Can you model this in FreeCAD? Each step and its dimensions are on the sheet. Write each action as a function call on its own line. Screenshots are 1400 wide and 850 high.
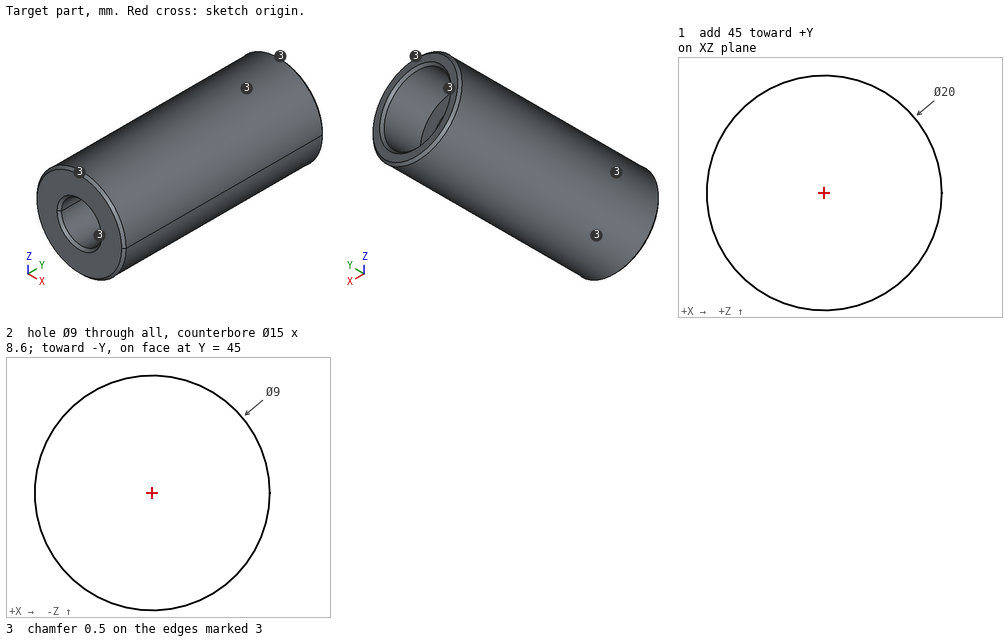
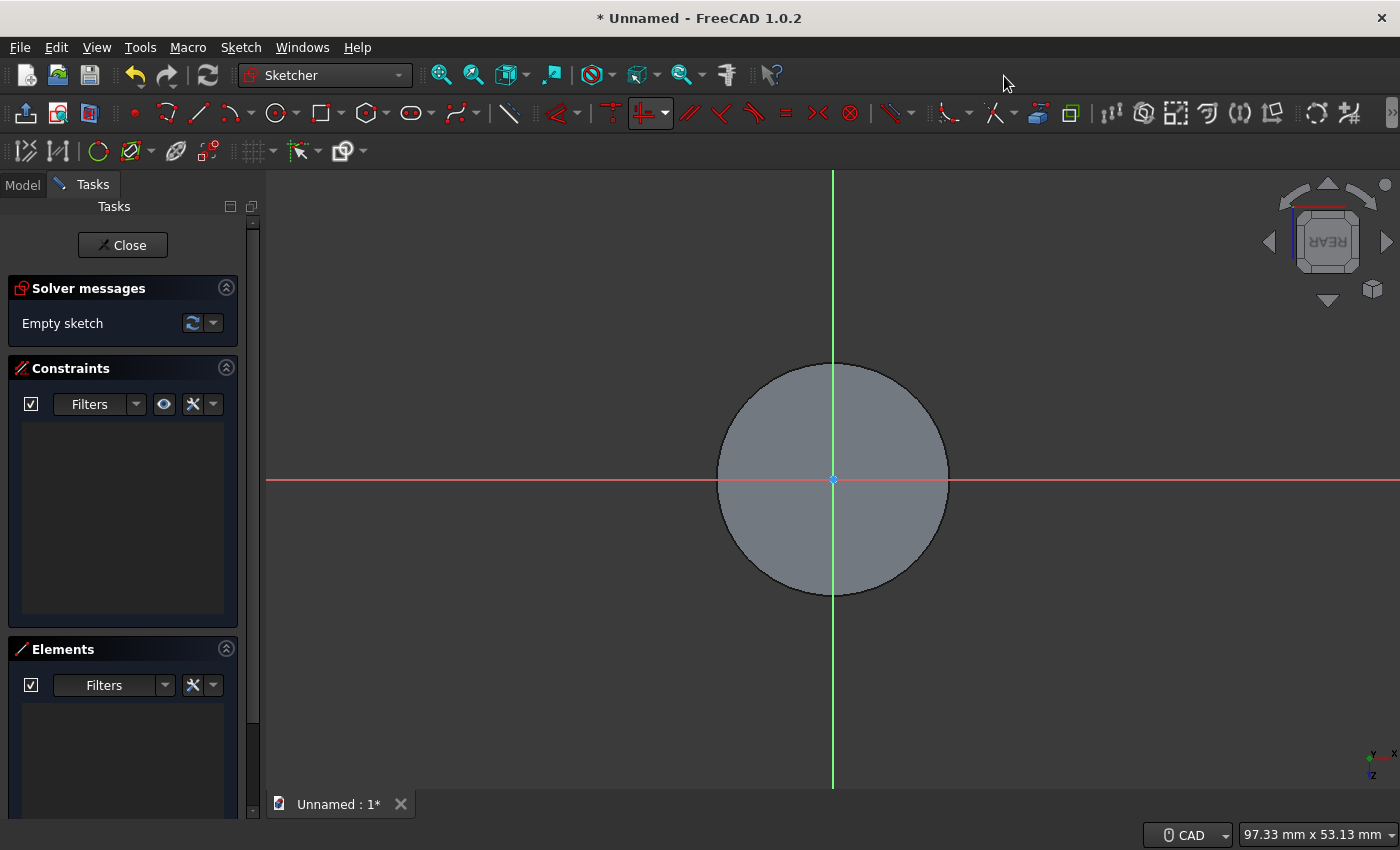
scroll(855, 479, up, 7)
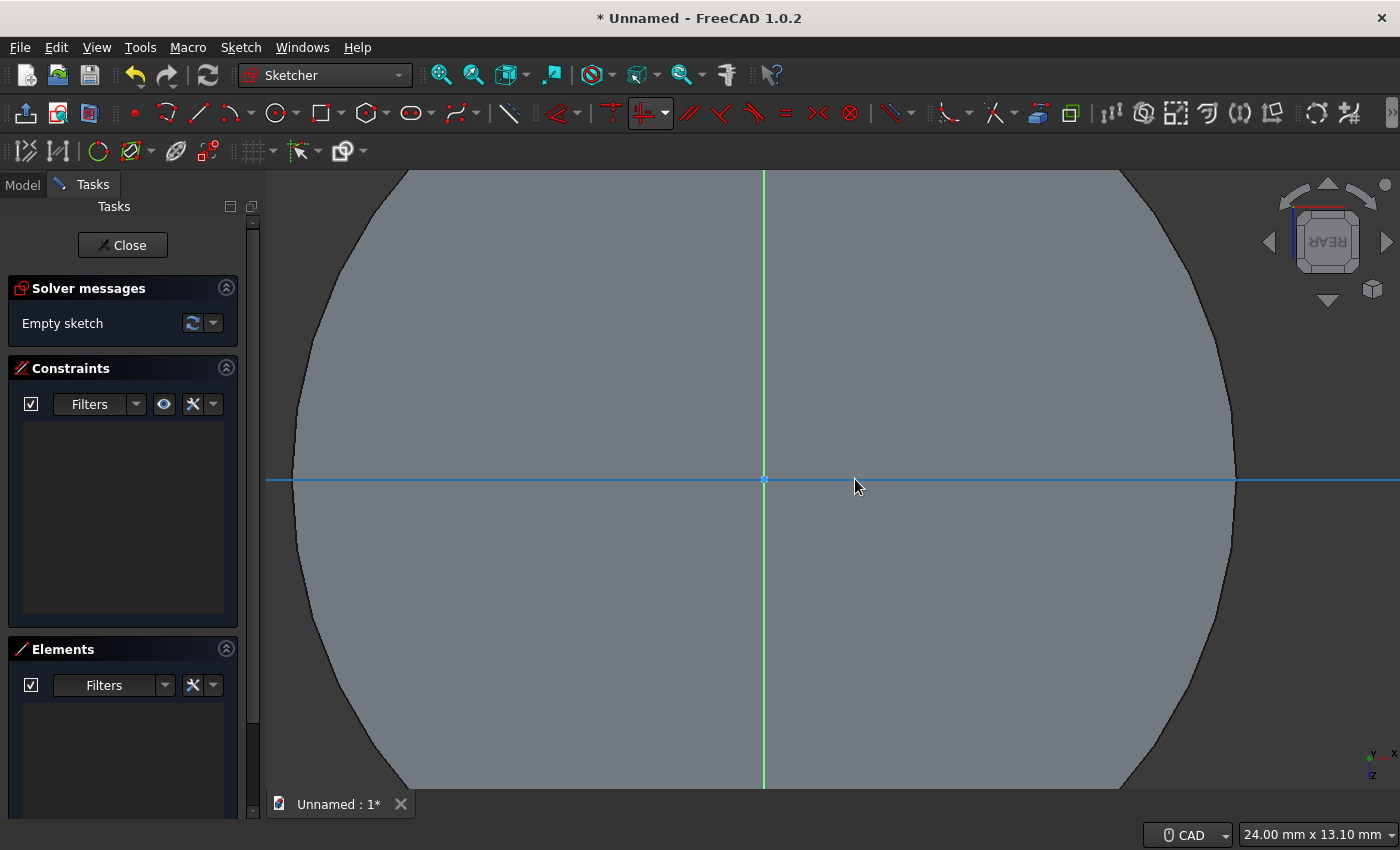
click(276, 114)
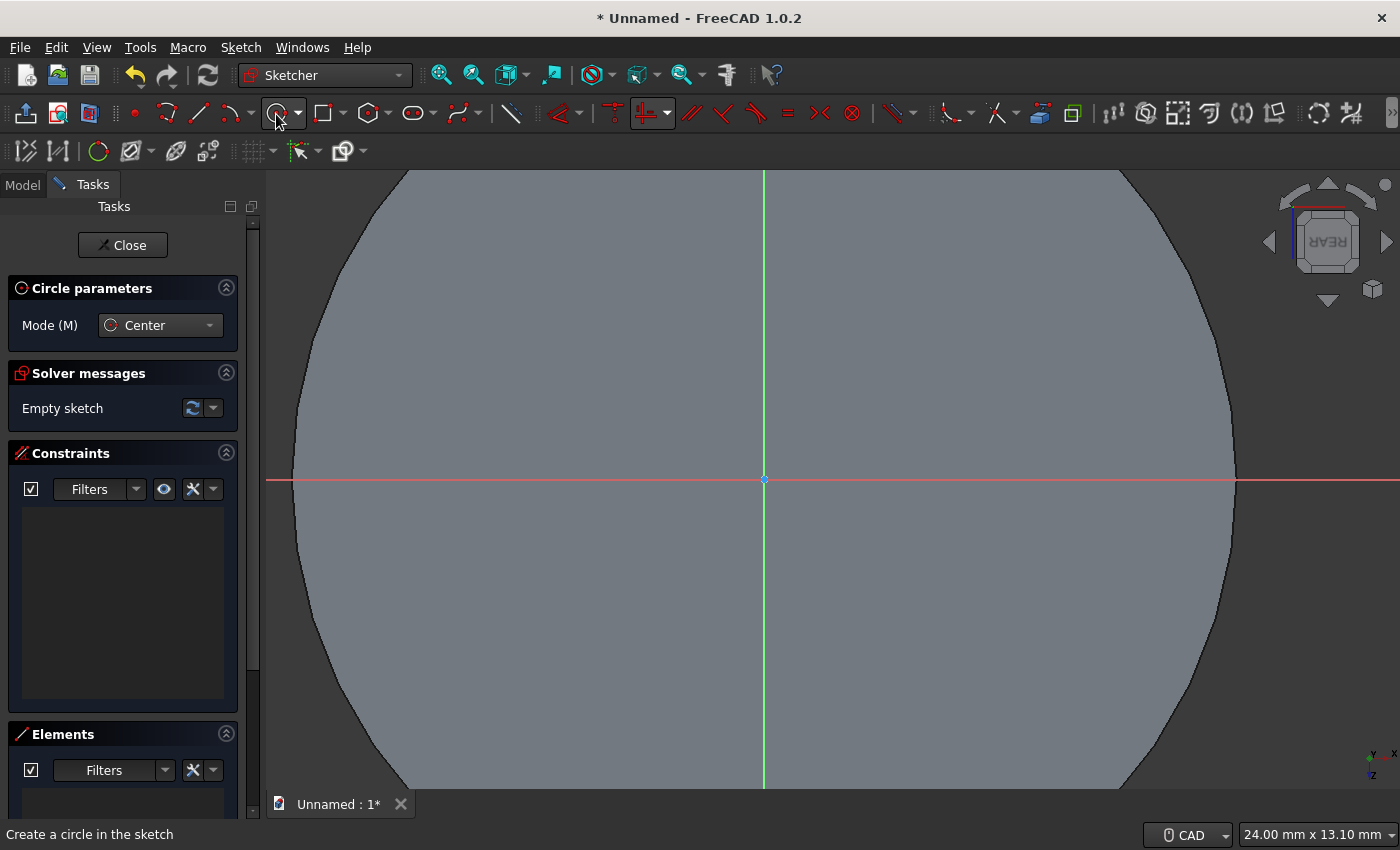
click(764, 479)
move(915, 329)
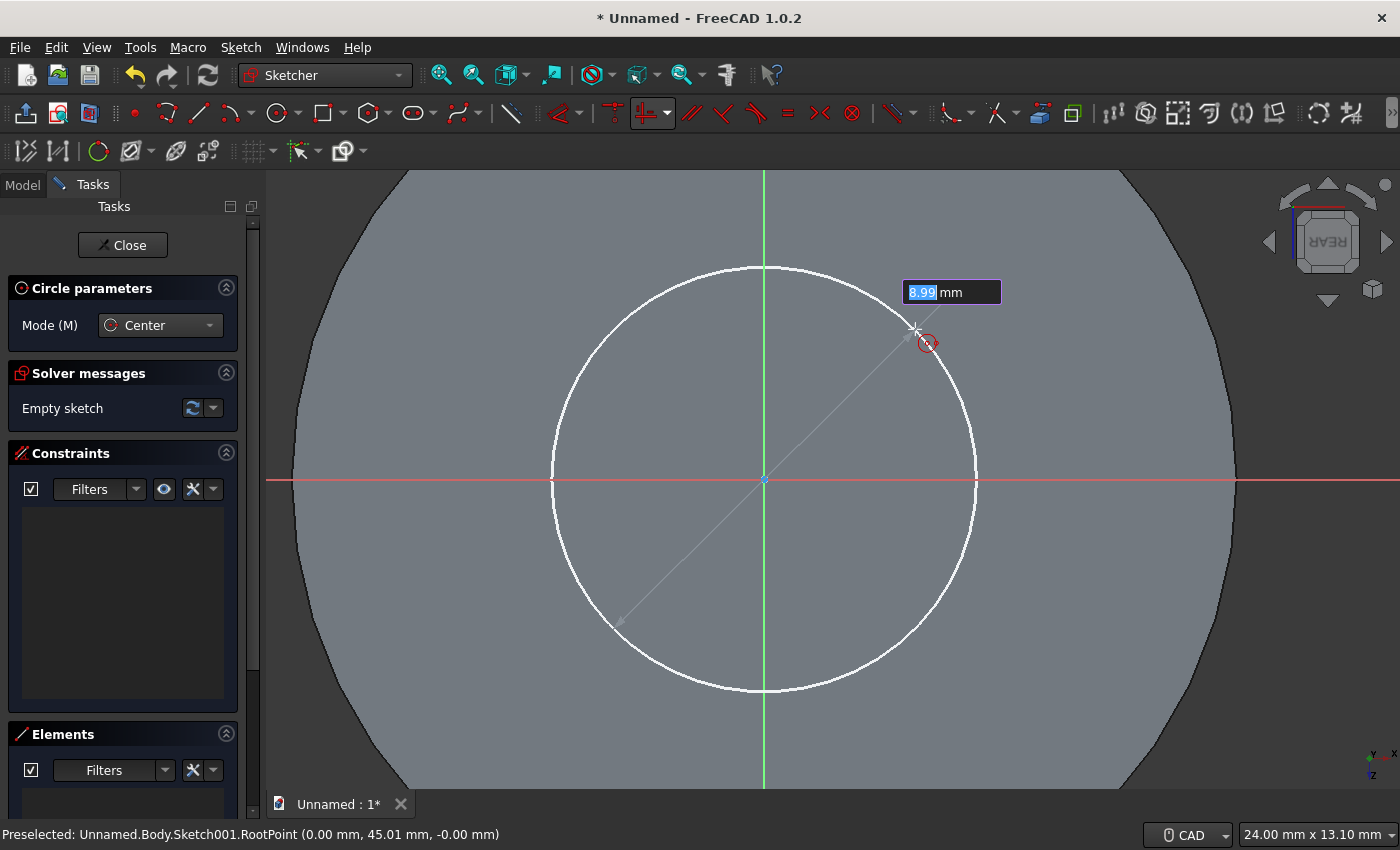
text(9)
key(Return)
key(Escape)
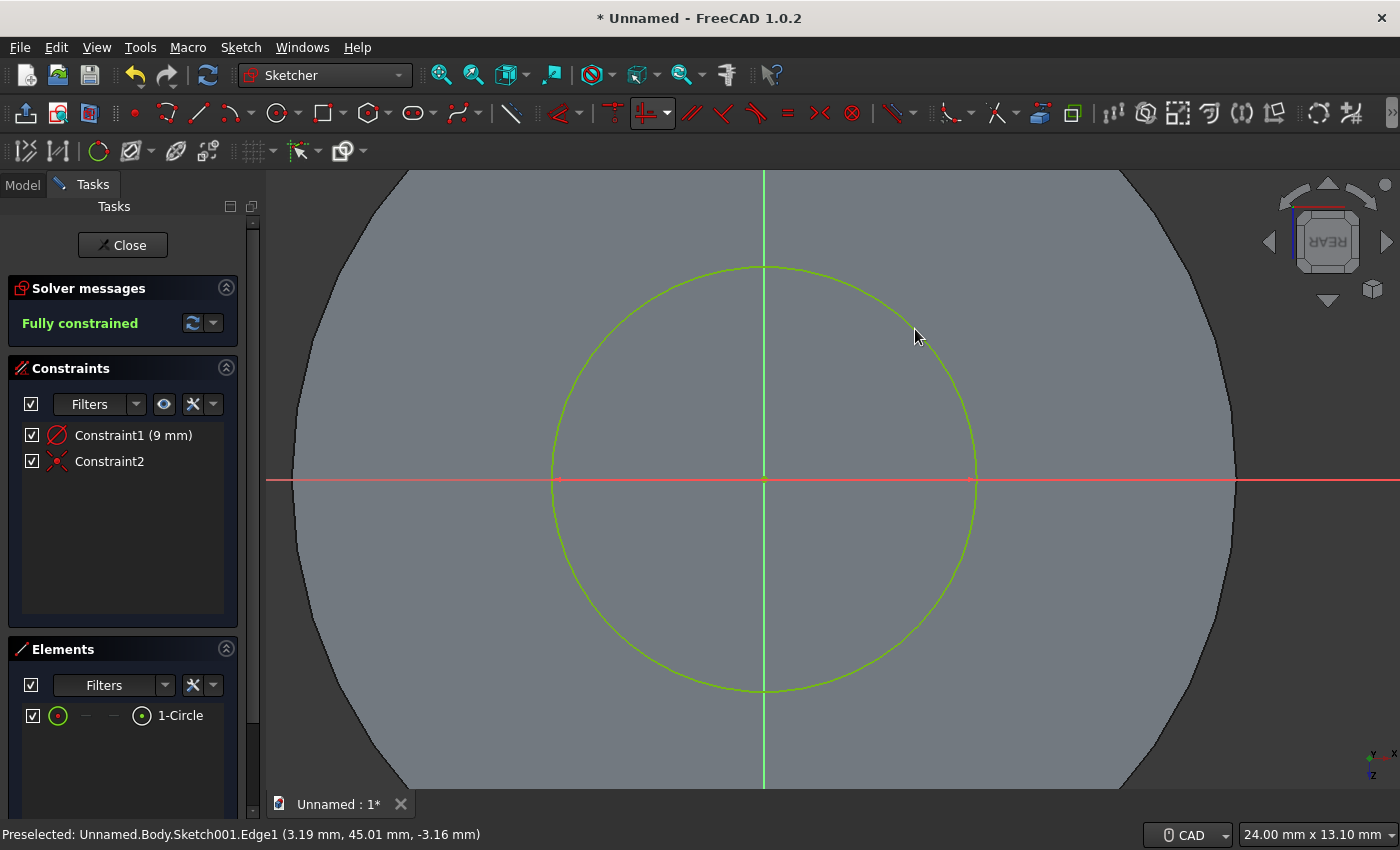
click(123, 245)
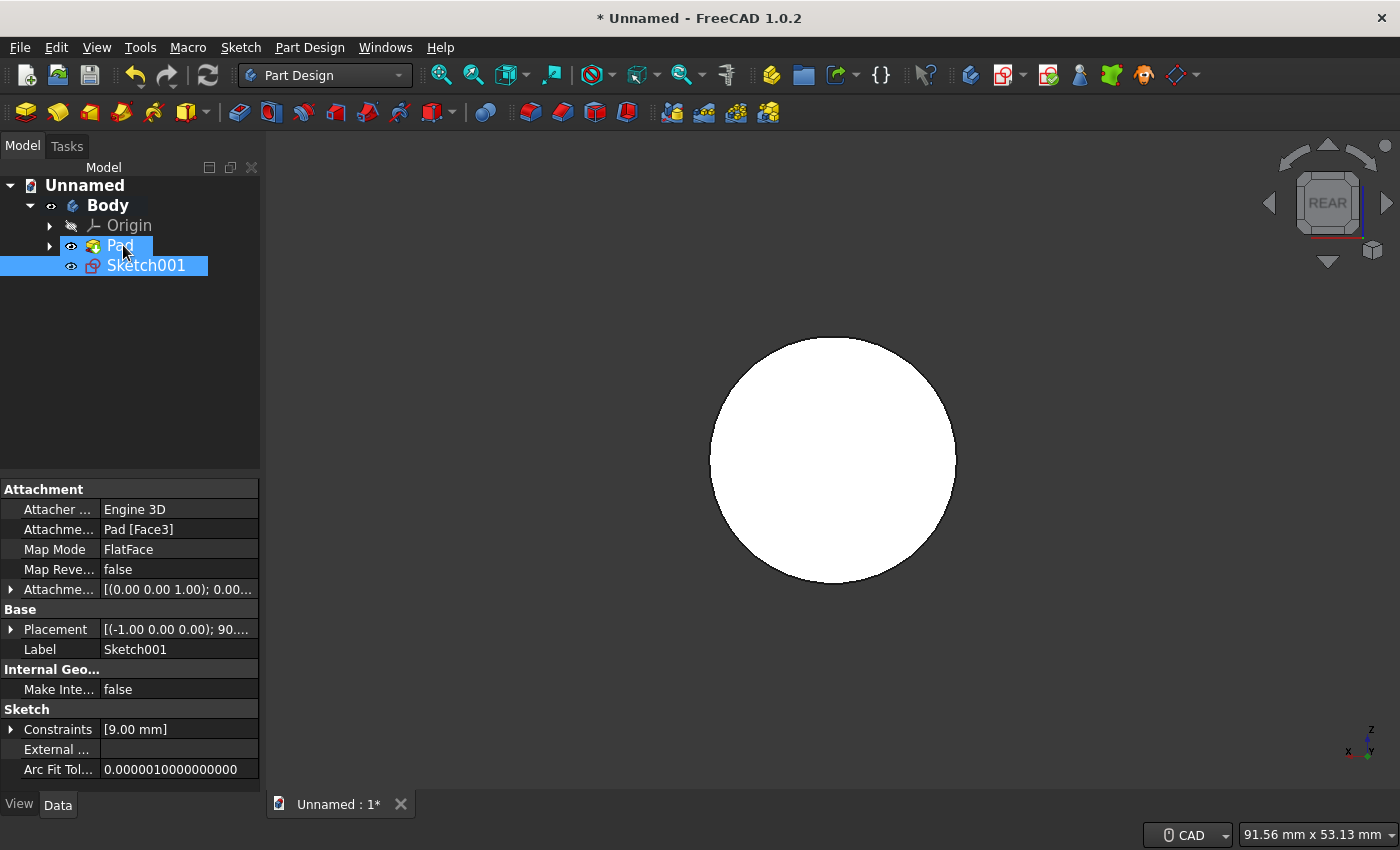
click(272, 112)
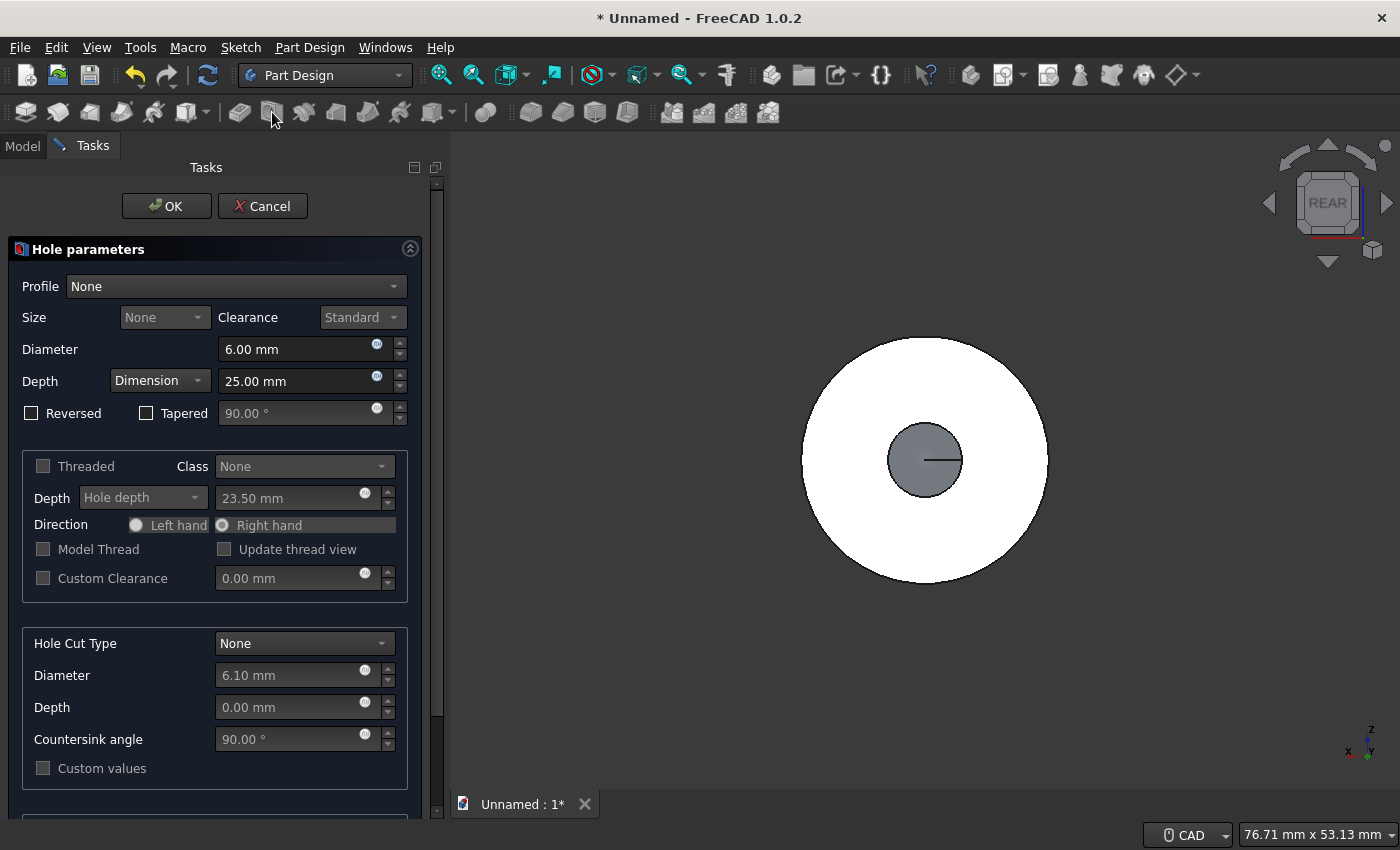
triple_click(305, 349)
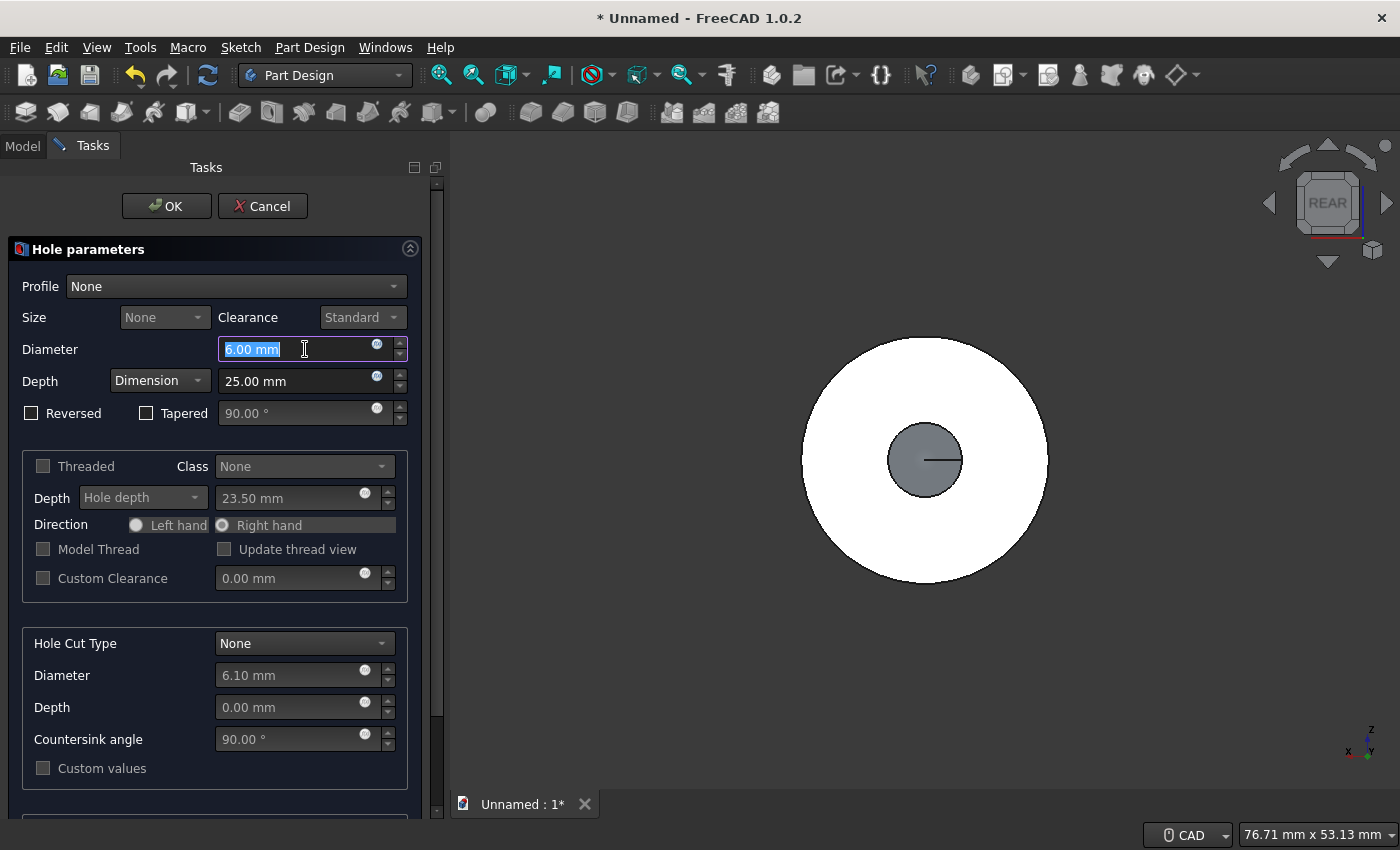
text(9)
key(Tab)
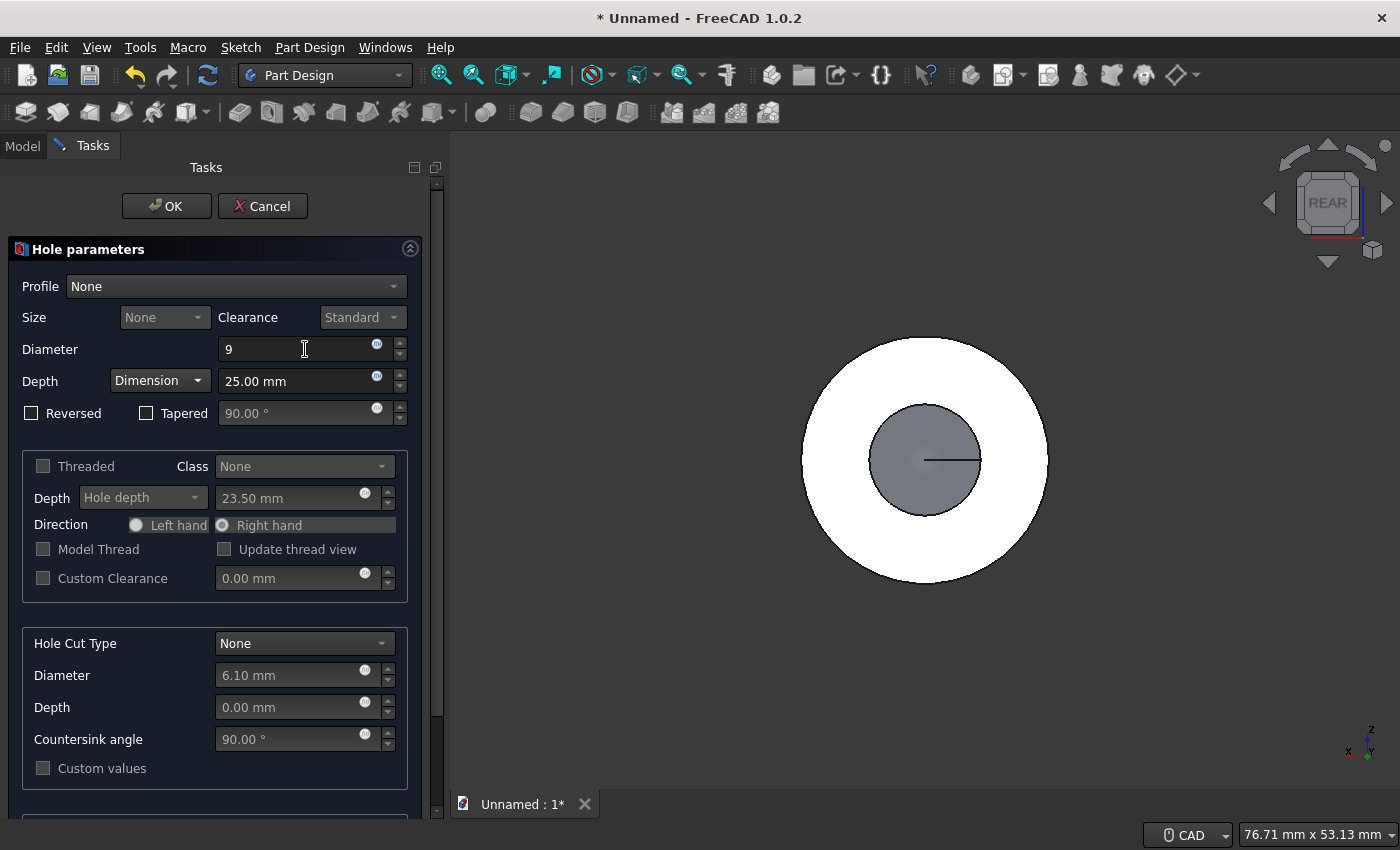
click(161, 380)